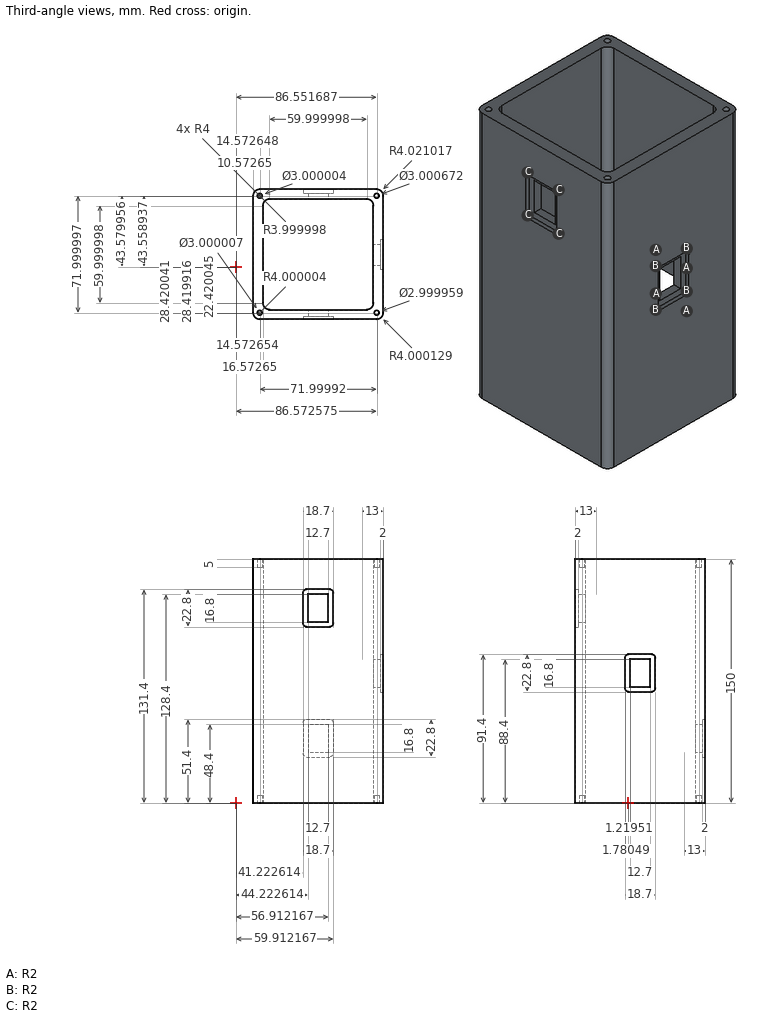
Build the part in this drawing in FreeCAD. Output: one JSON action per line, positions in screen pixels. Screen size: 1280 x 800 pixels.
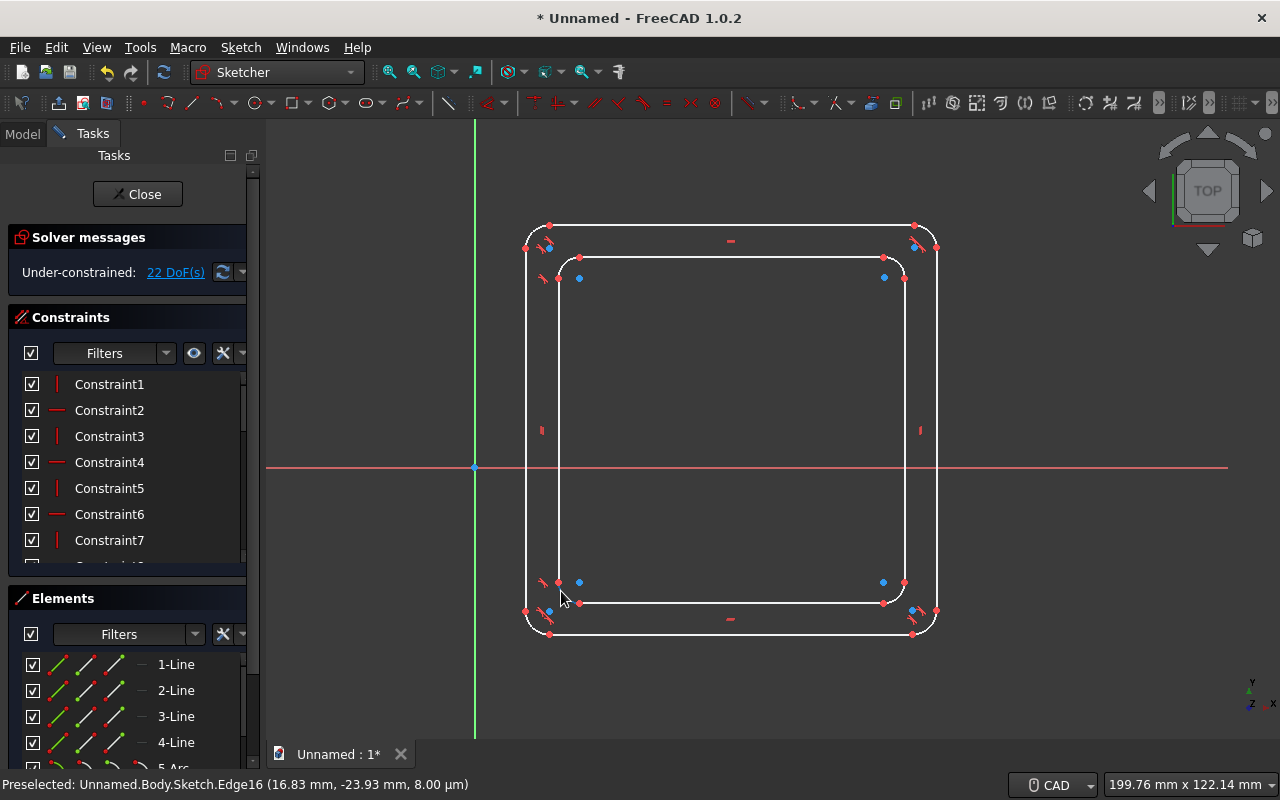
{"action": "left_click", "coordinate": [671, 257]}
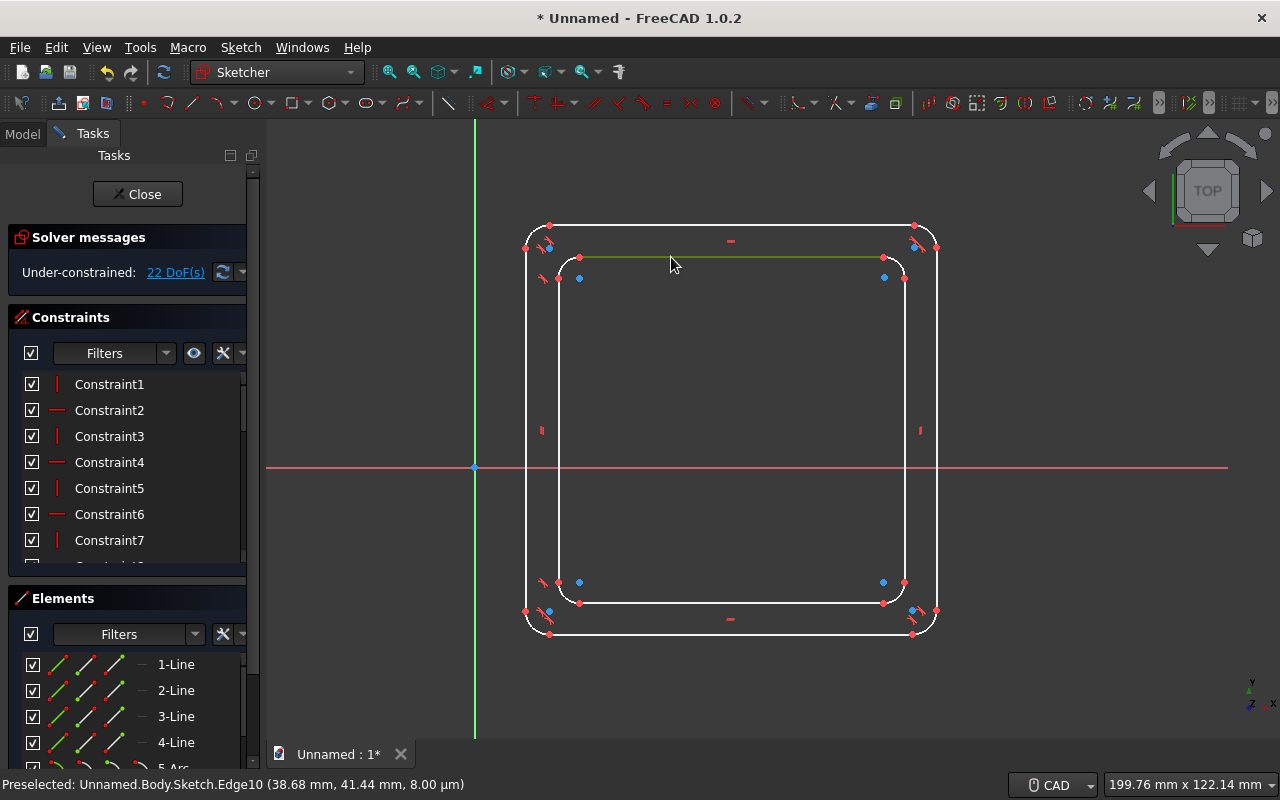
{"action": "scroll", "coordinate": [570, 260], "scroll_direction": "up", "scroll_amount": 2}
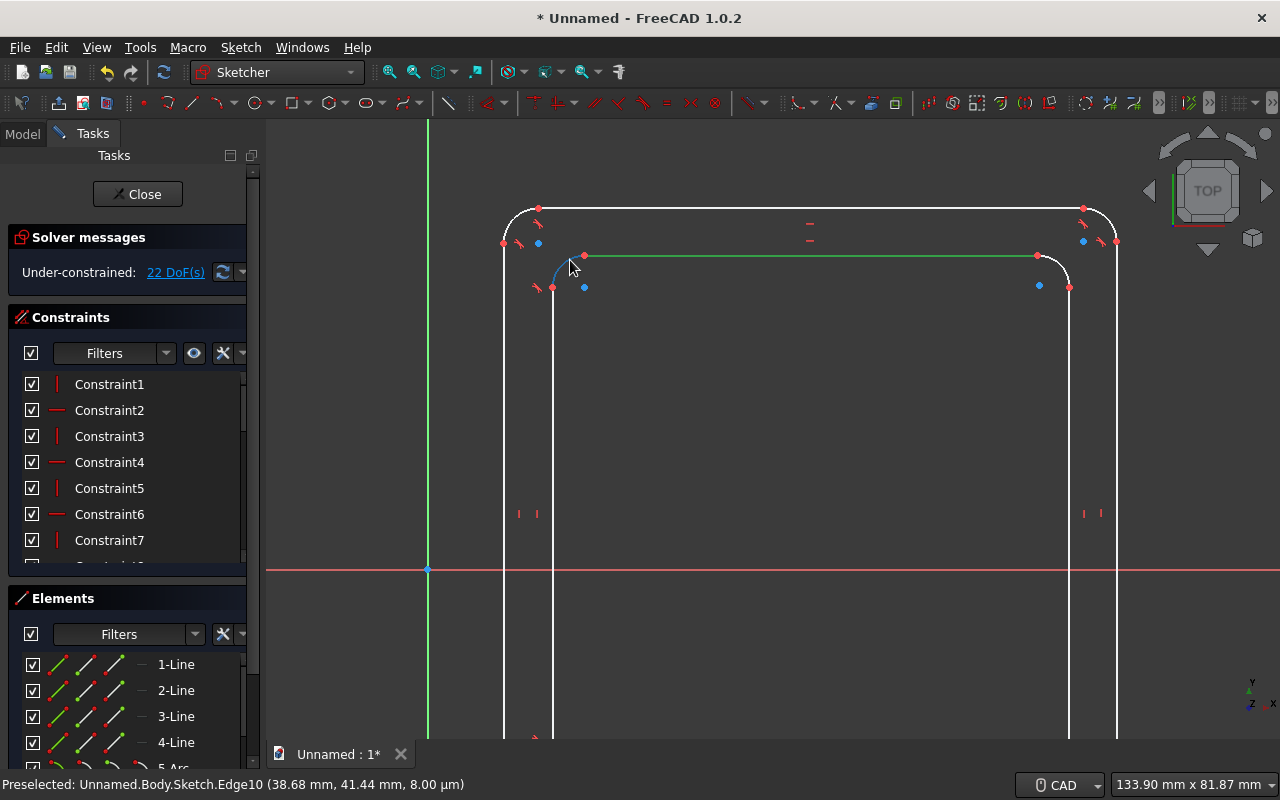
{"action": "left_click", "coordinate": [570, 259]}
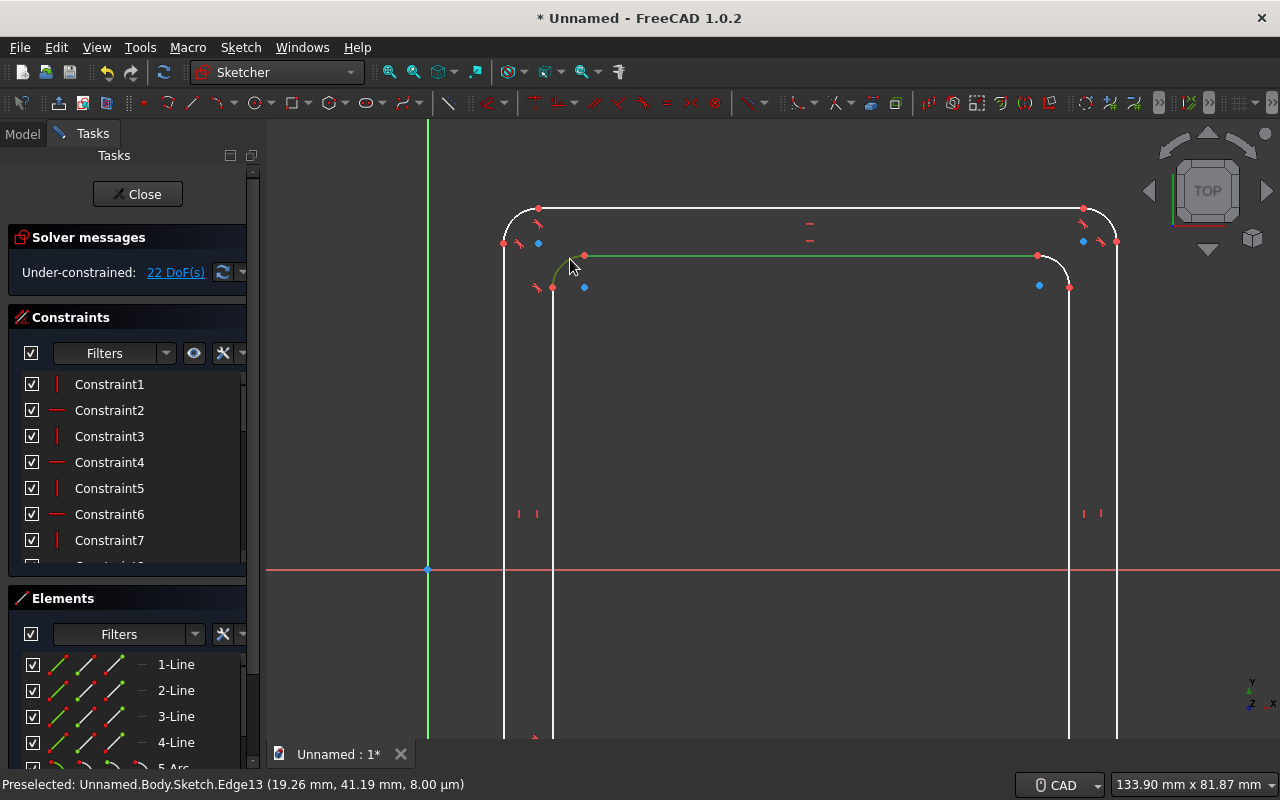
{"action": "left_click", "coordinate": [644, 104]}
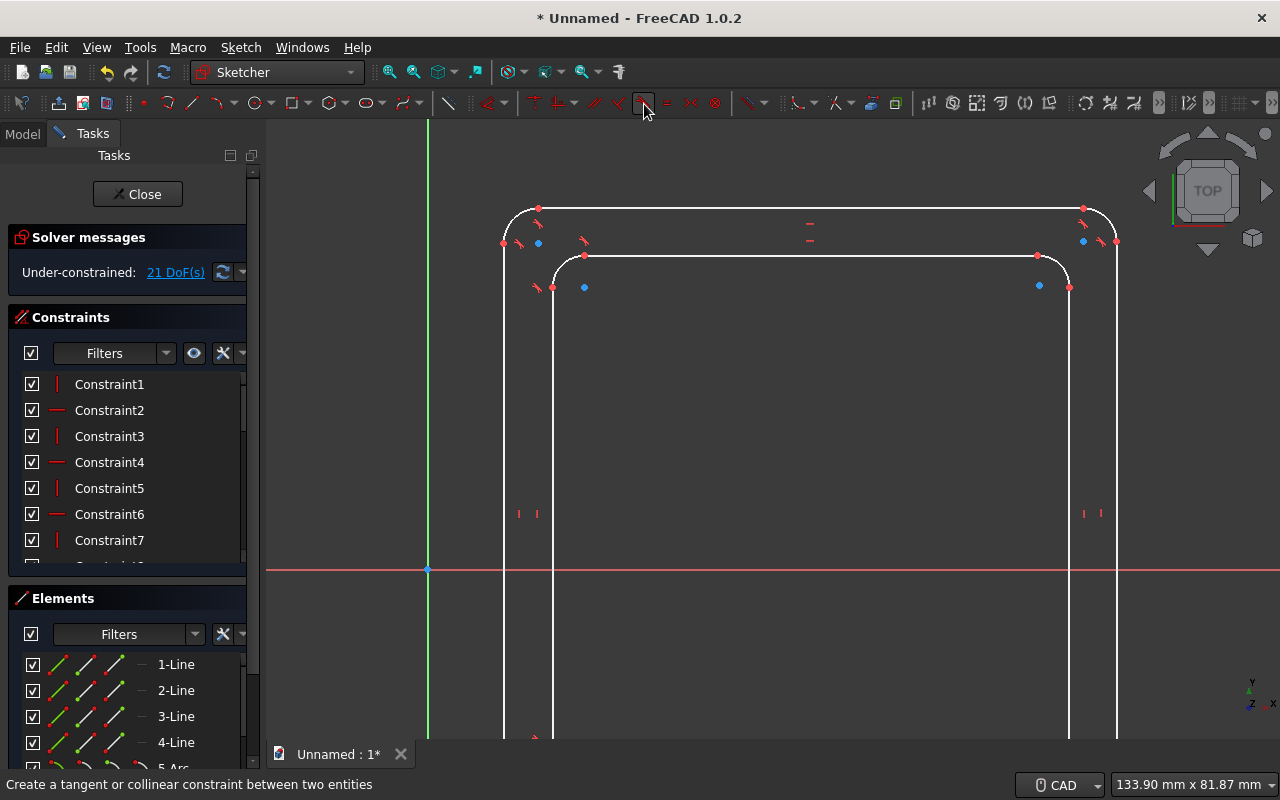
{"action": "left_click", "coordinate": [720, 256]}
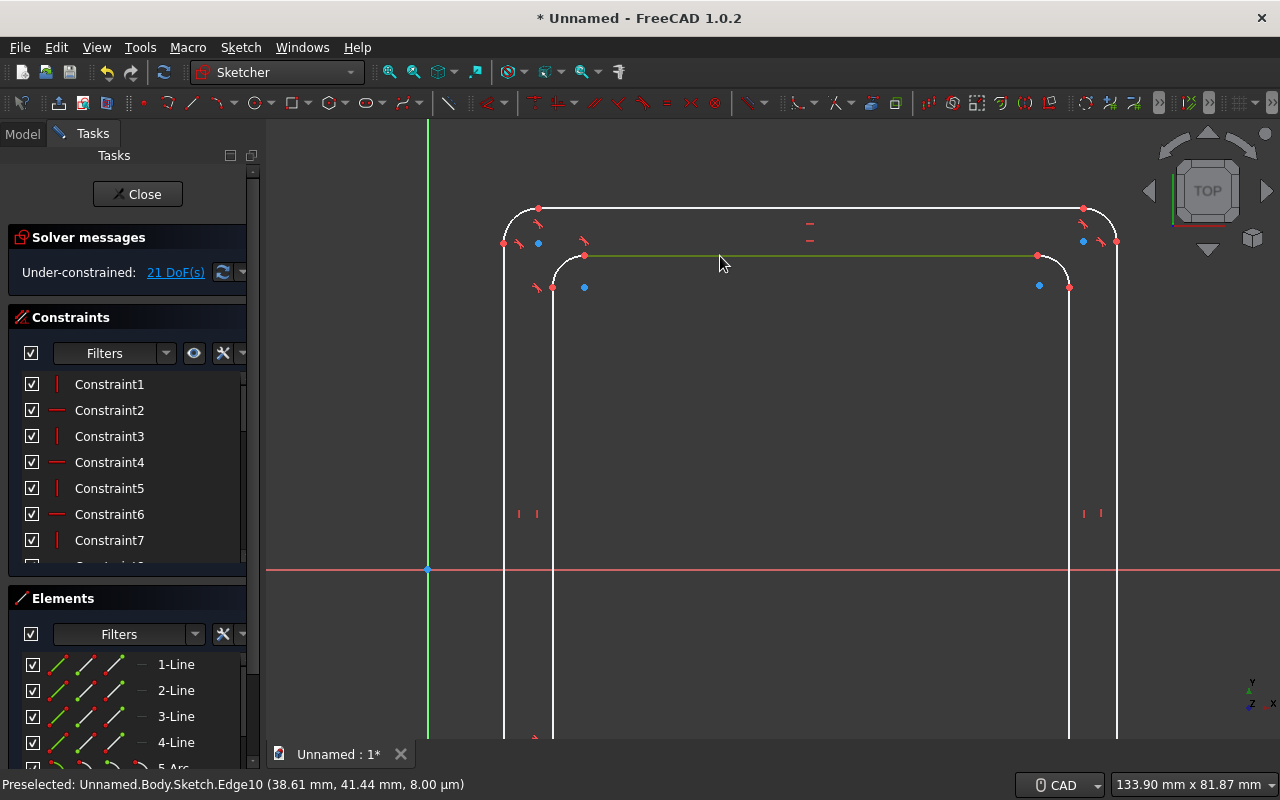
{"action": "left_click", "coordinate": [1066, 273]}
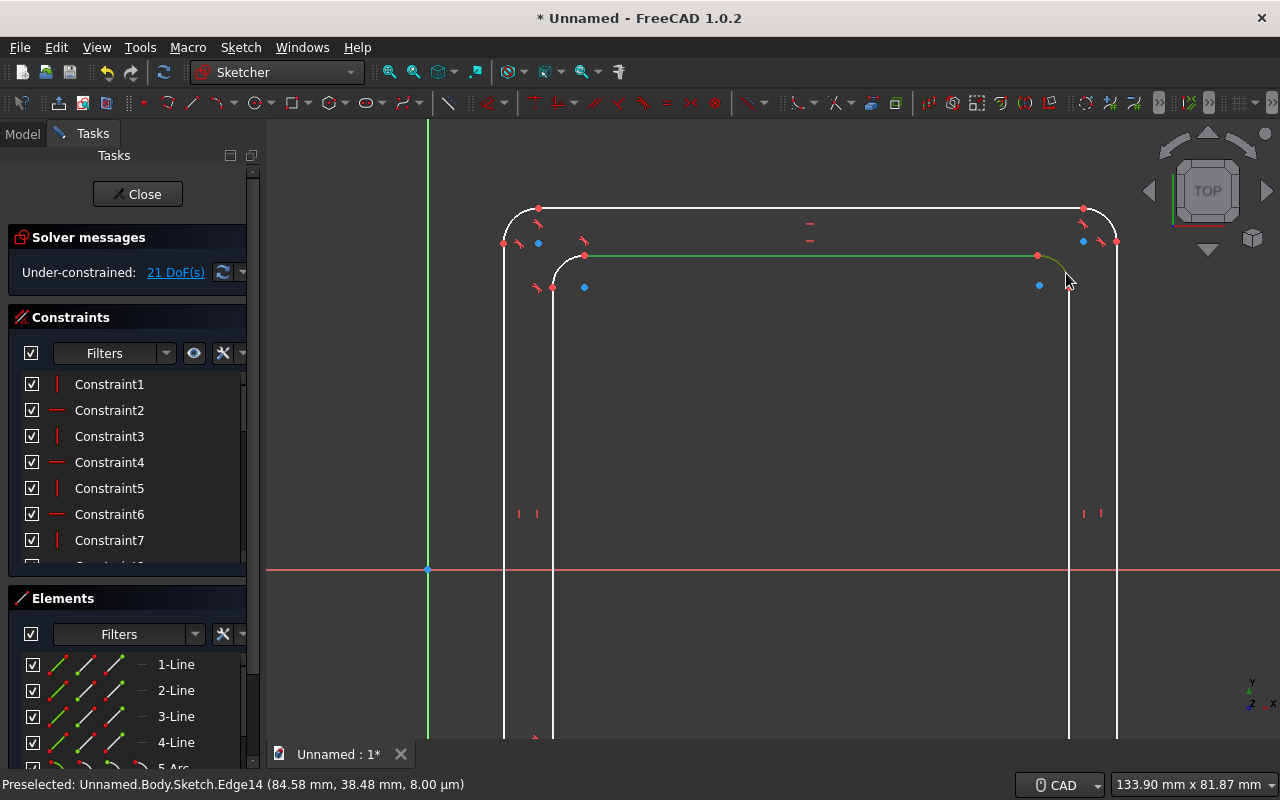
{"action": "left_click", "coordinate": [644, 104]}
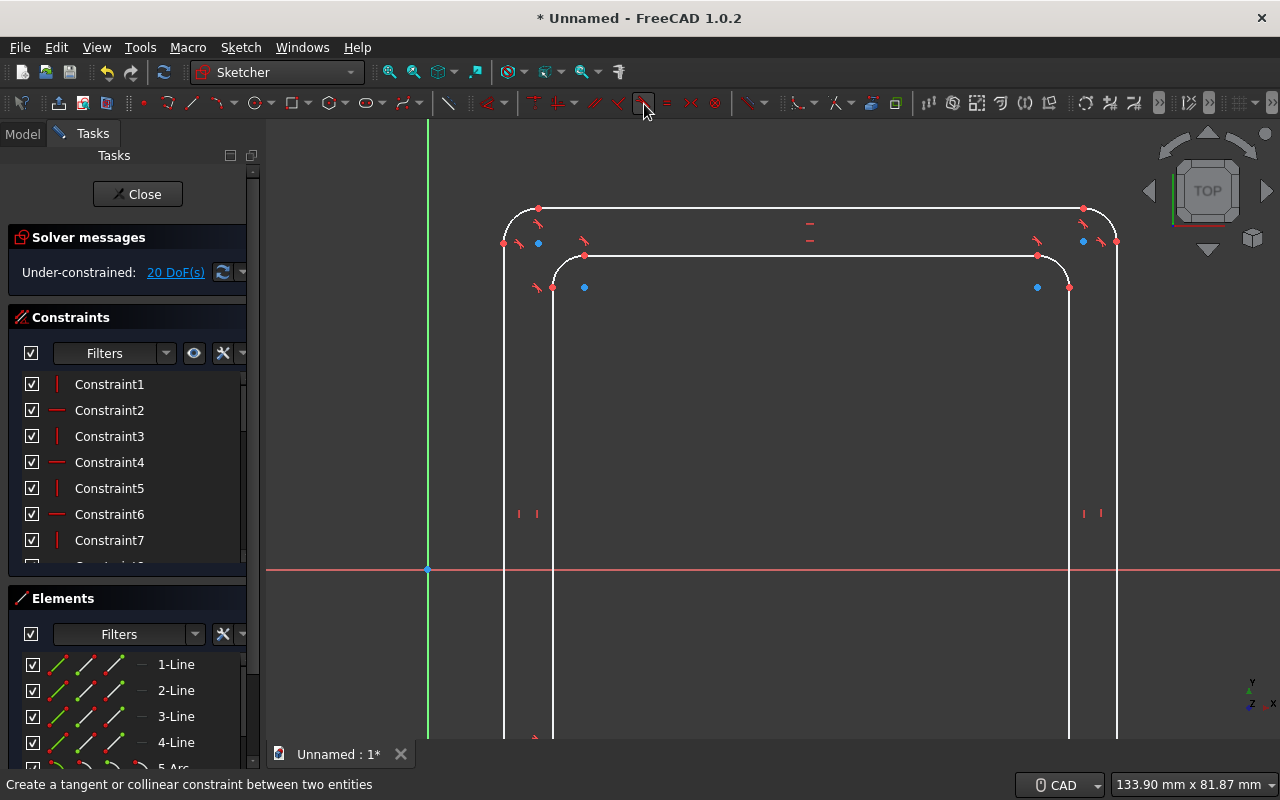
{"action": "left_click", "coordinate": [1069, 423]}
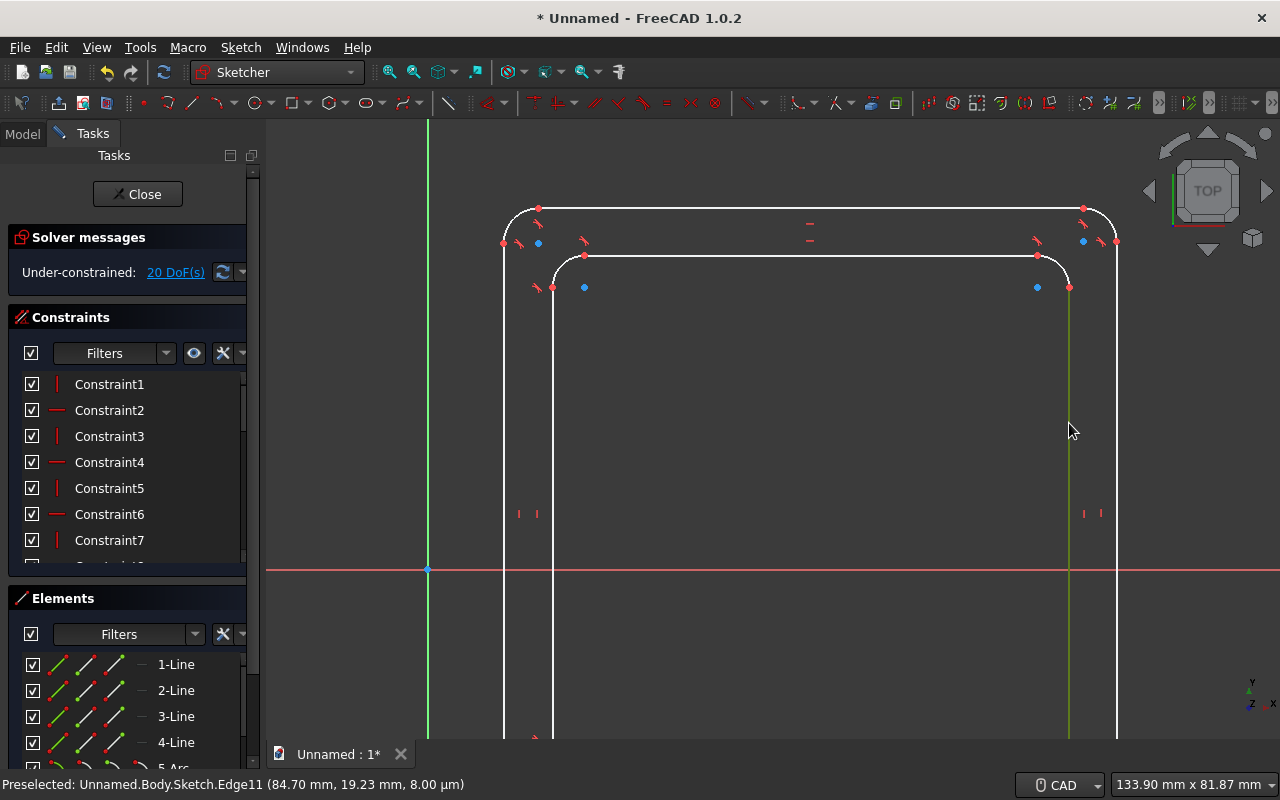
{"action": "left_click", "coordinate": [1066, 273]}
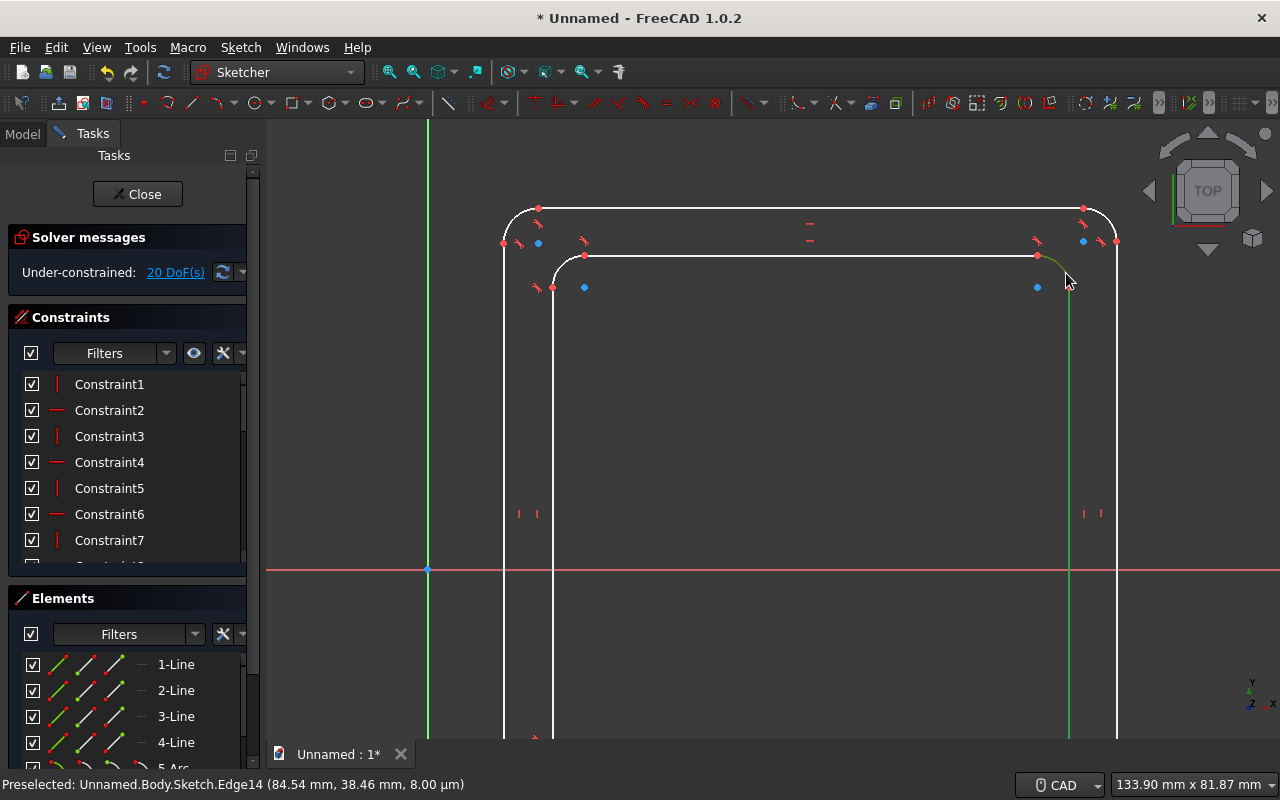
{"action": "left_click", "coordinate": [644, 104]}